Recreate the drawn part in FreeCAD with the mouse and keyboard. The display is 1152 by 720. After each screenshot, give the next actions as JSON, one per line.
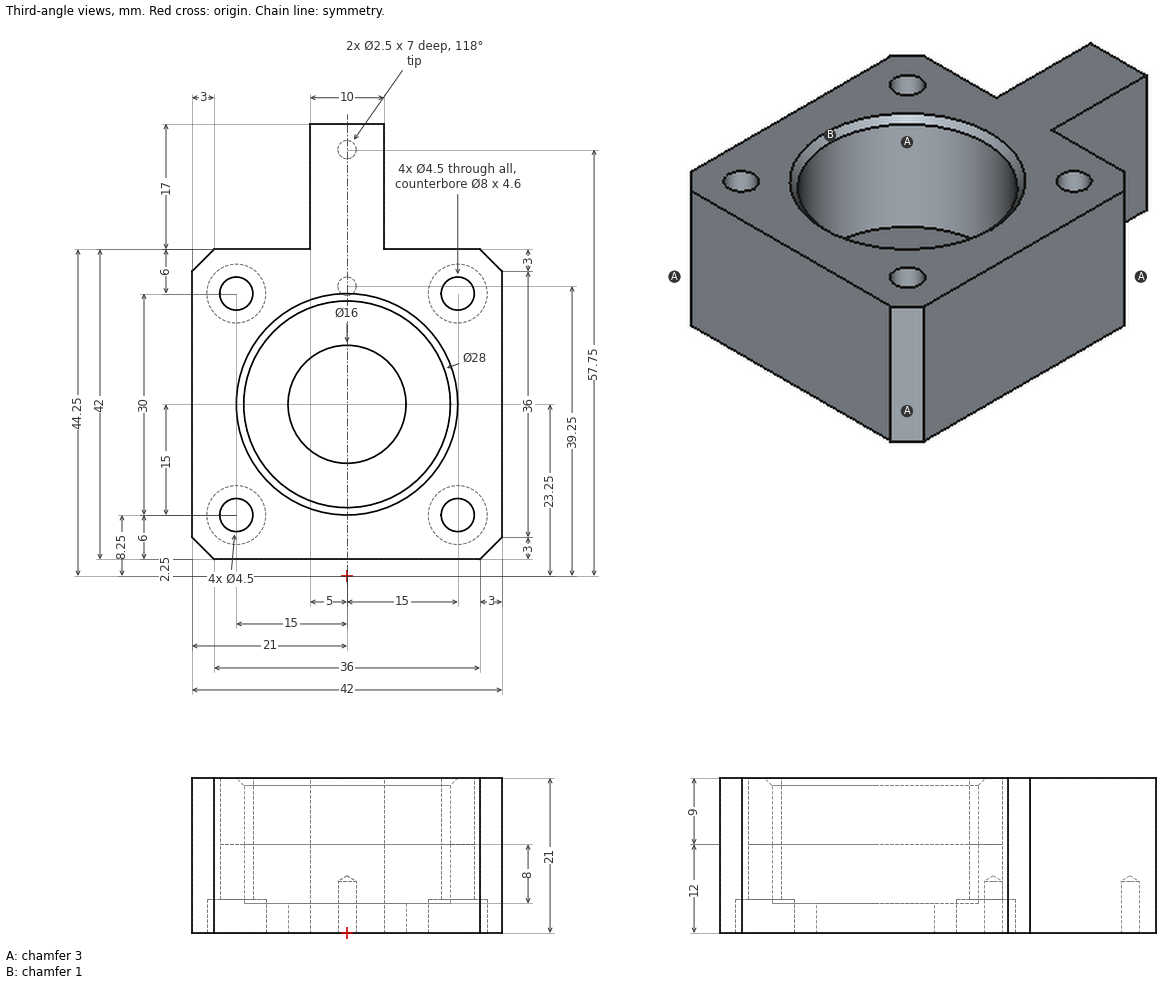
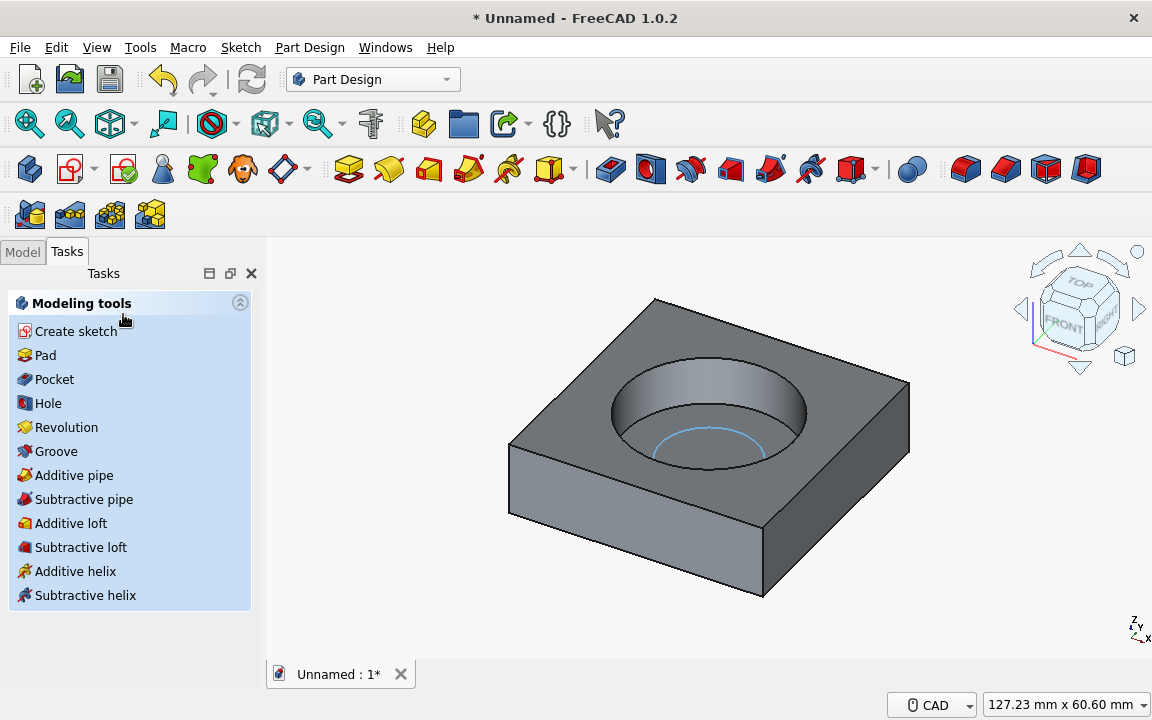
{"action": "left_click", "coordinate": [612, 170]}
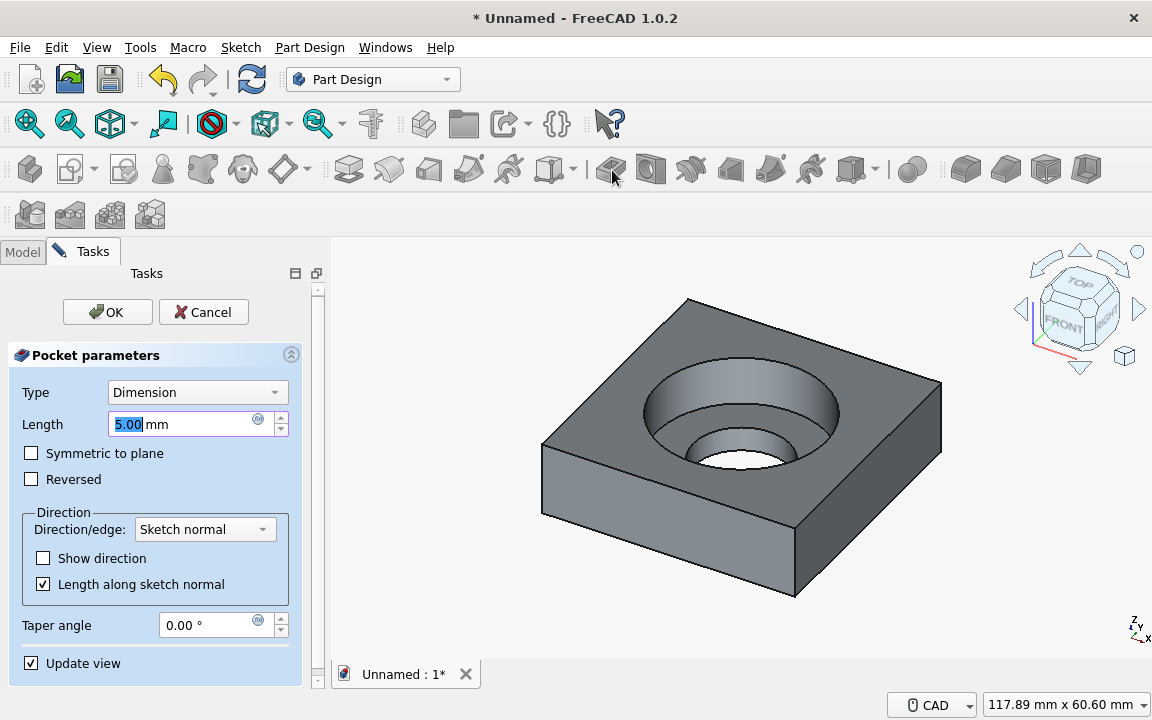
{"action": "left_click", "coordinate": [198, 392]}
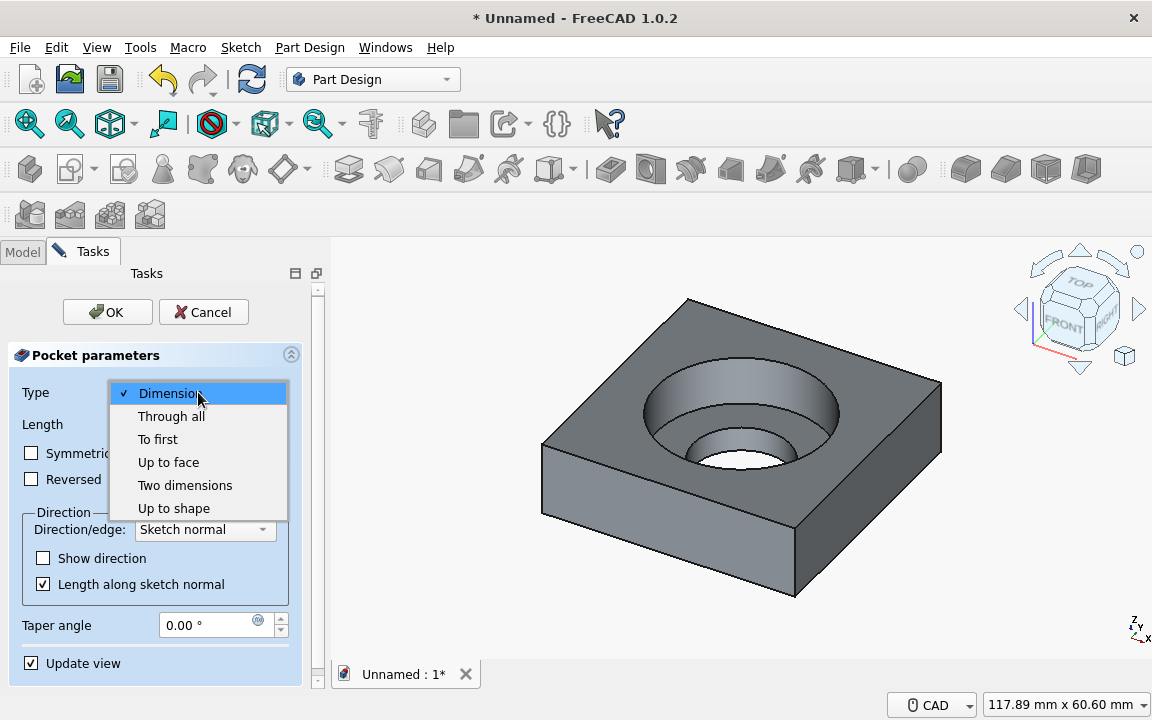
{"action": "left_click", "coordinate": [198, 416]}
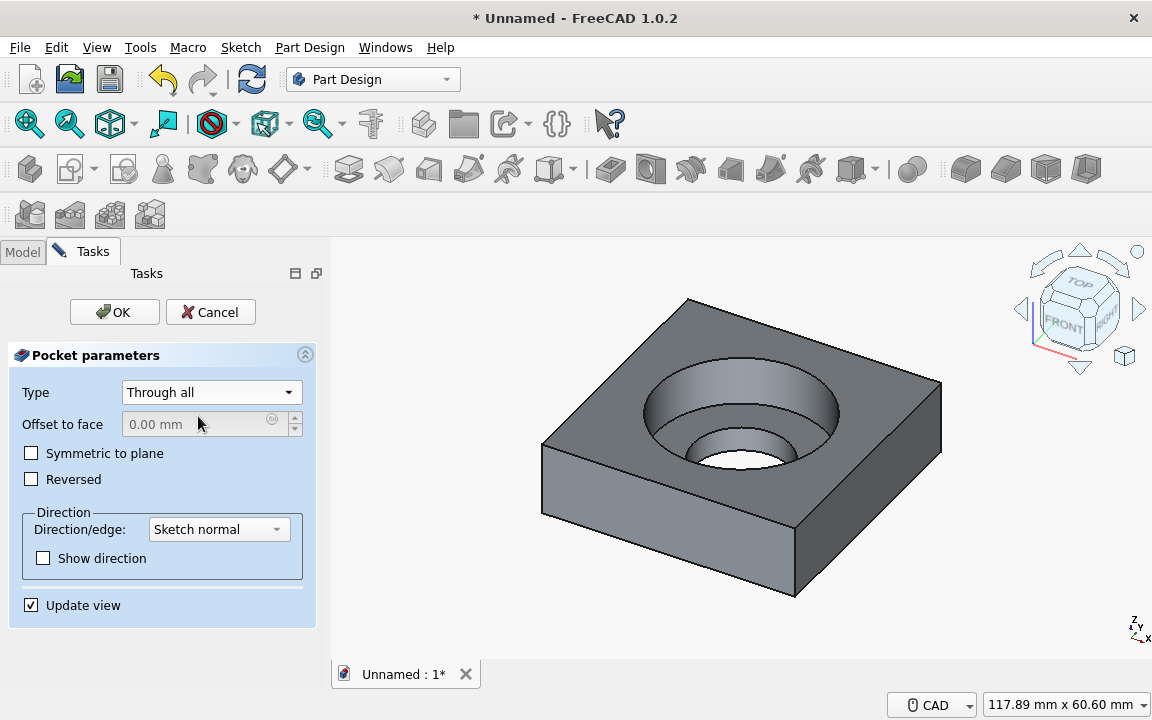
{"action": "left_click", "coordinate": [115, 312]}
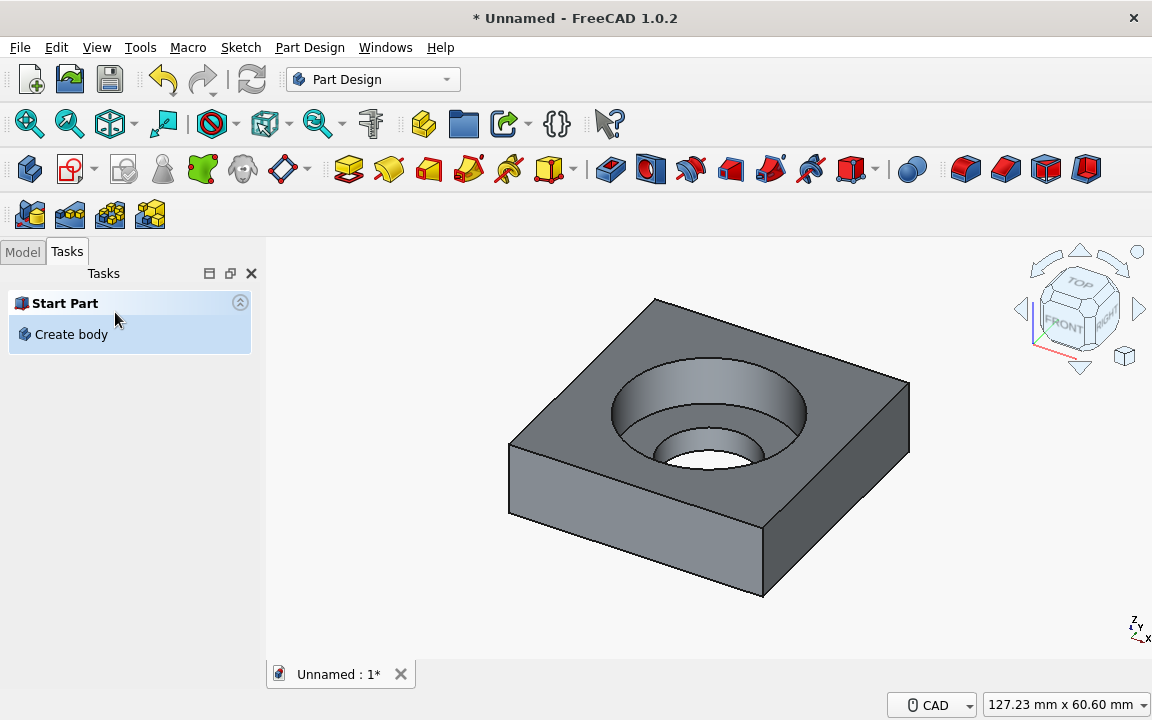
{"action": "left_click", "coordinate": [763, 562]}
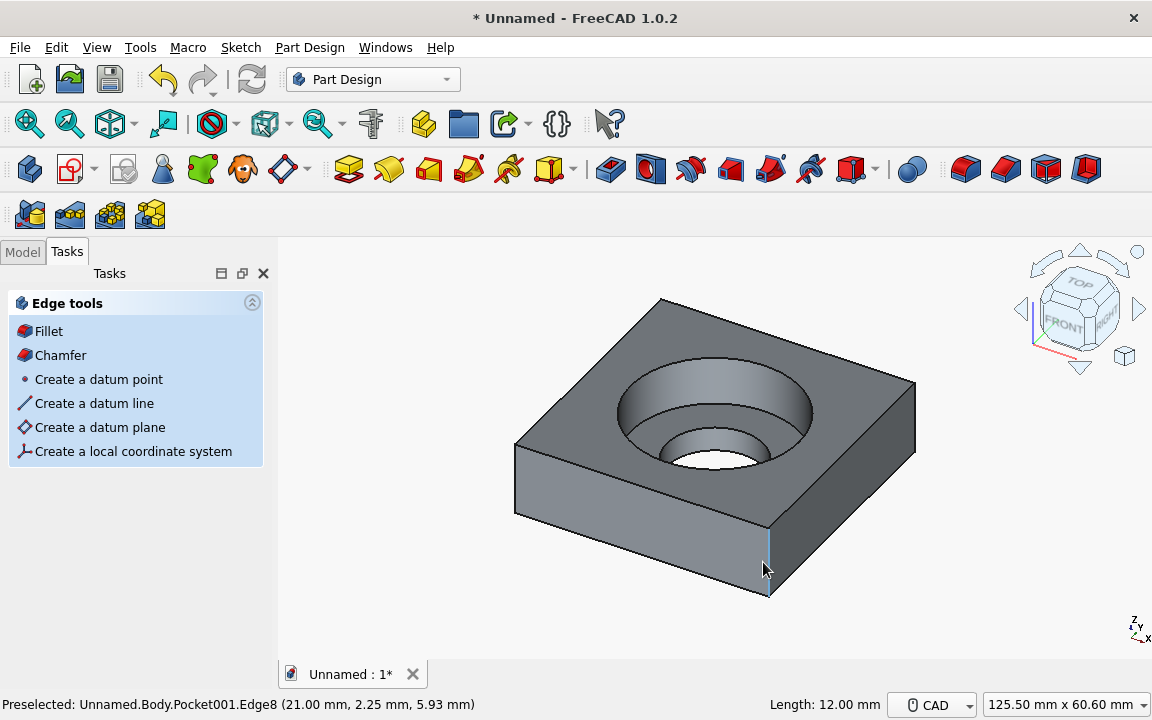
{"action": "key", "text": "0"}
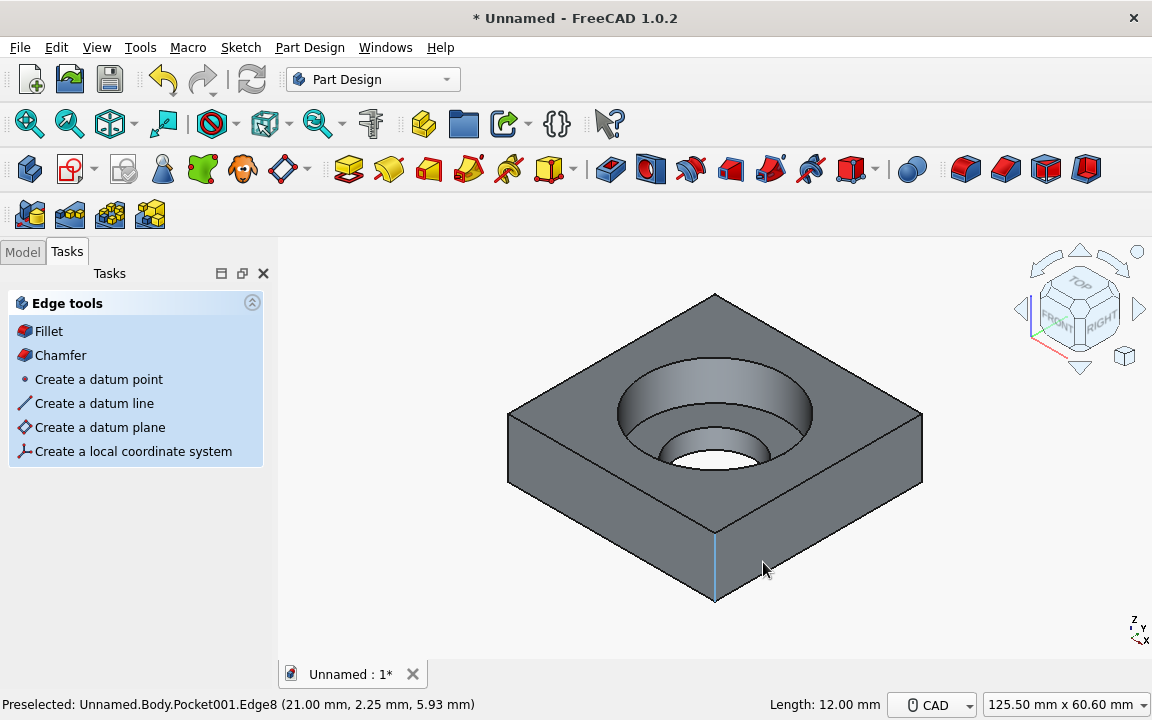
{"action": "key", "text": "2"}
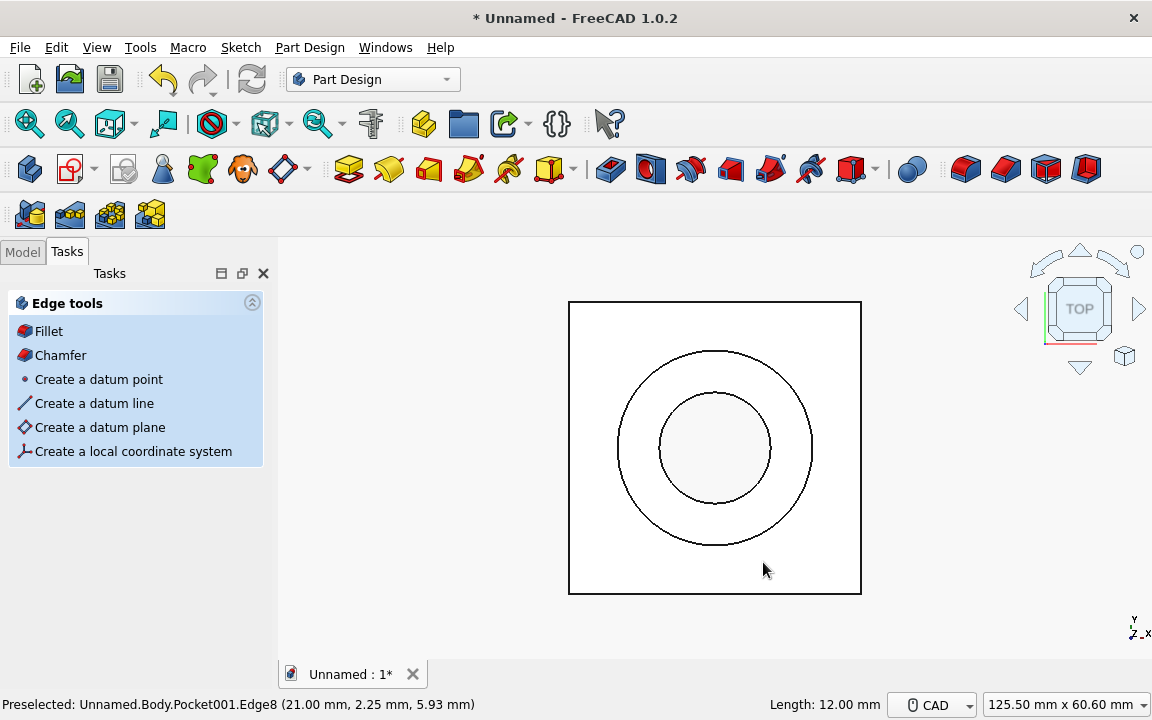
{"action": "key", "text": "1"}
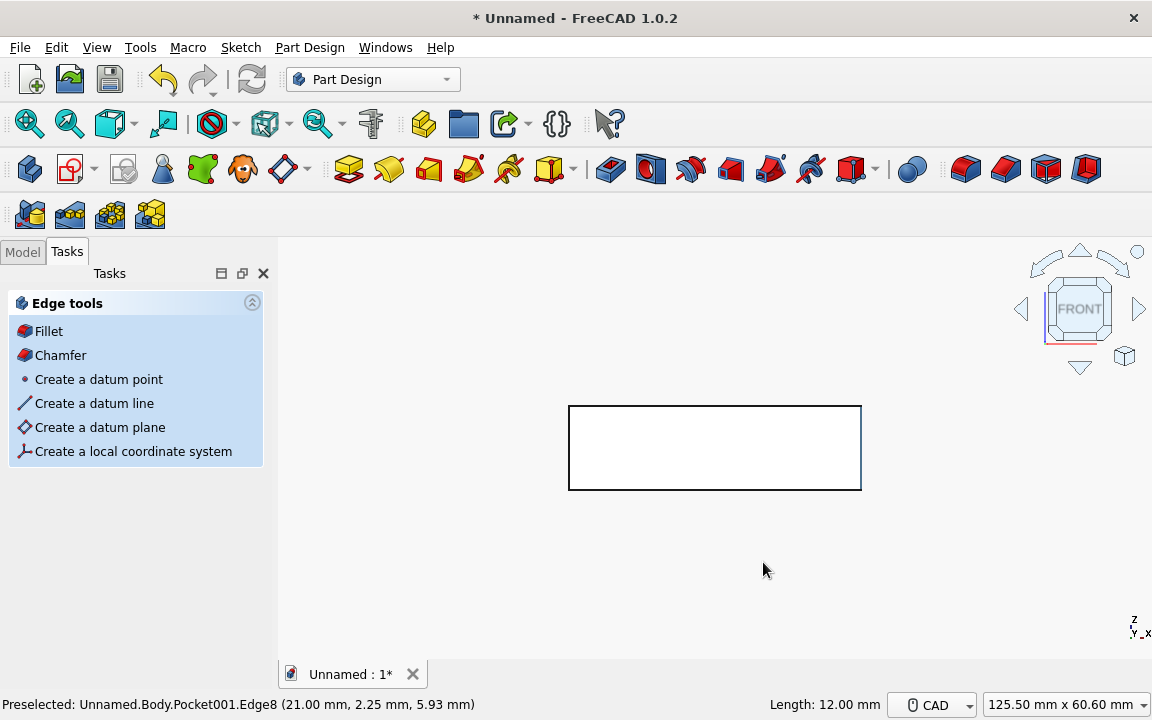
{"action": "left_click", "coordinate": [30, 124]}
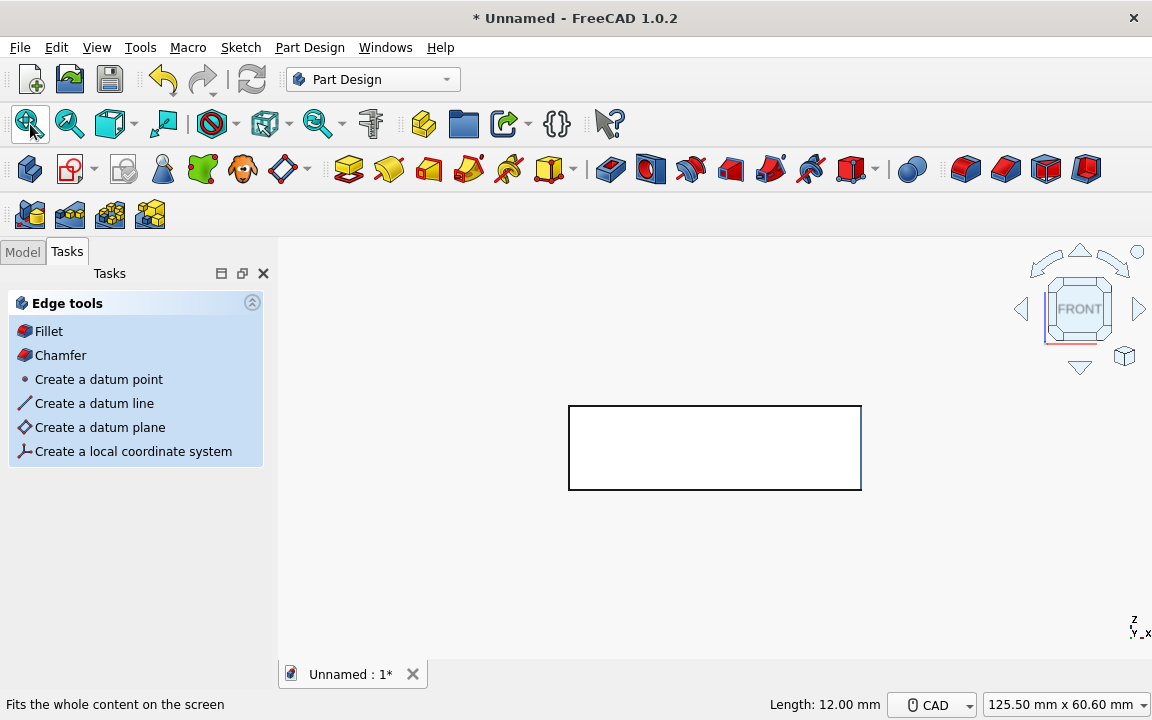
{"action": "left_click", "coordinate": [569, 447], "text": "ctrl"}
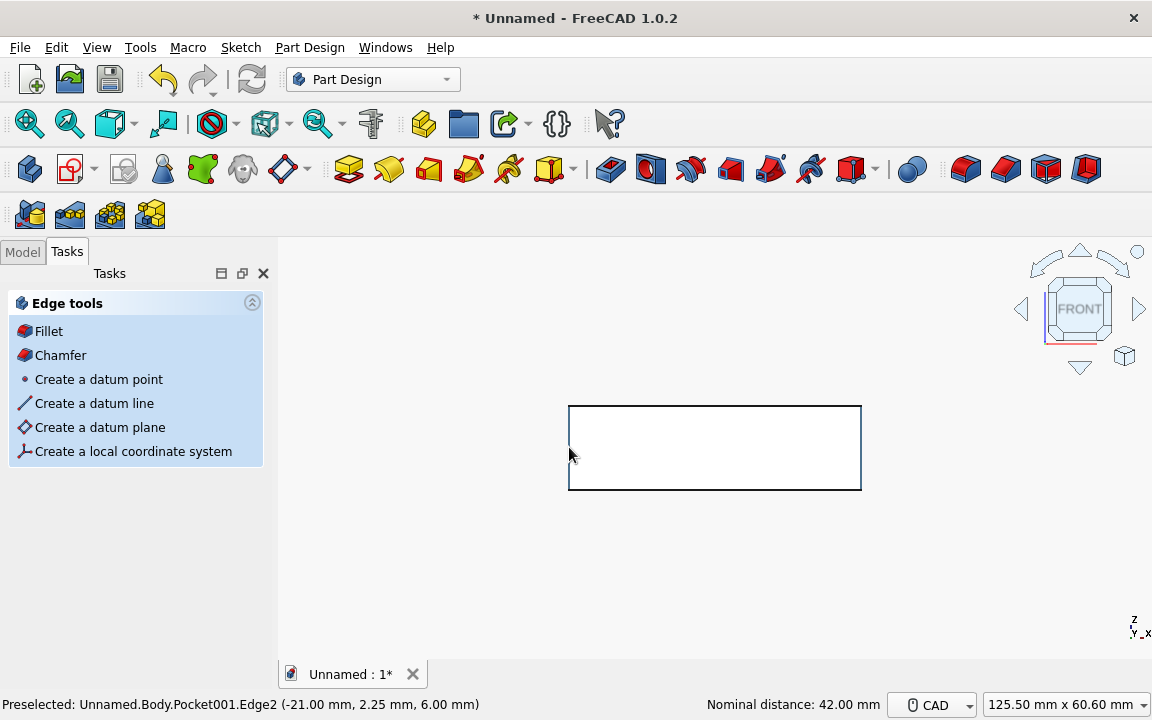
{"action": "key", "text": "3"}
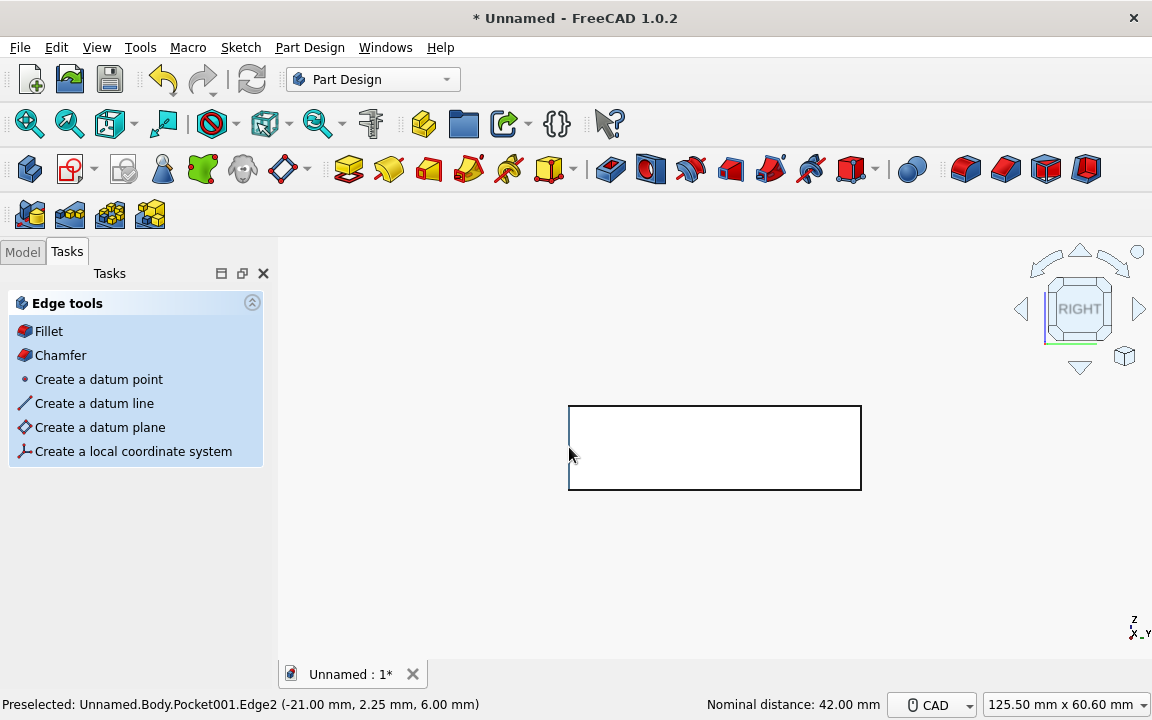
{"action": "left_click", "coordinate": [30, 124]}